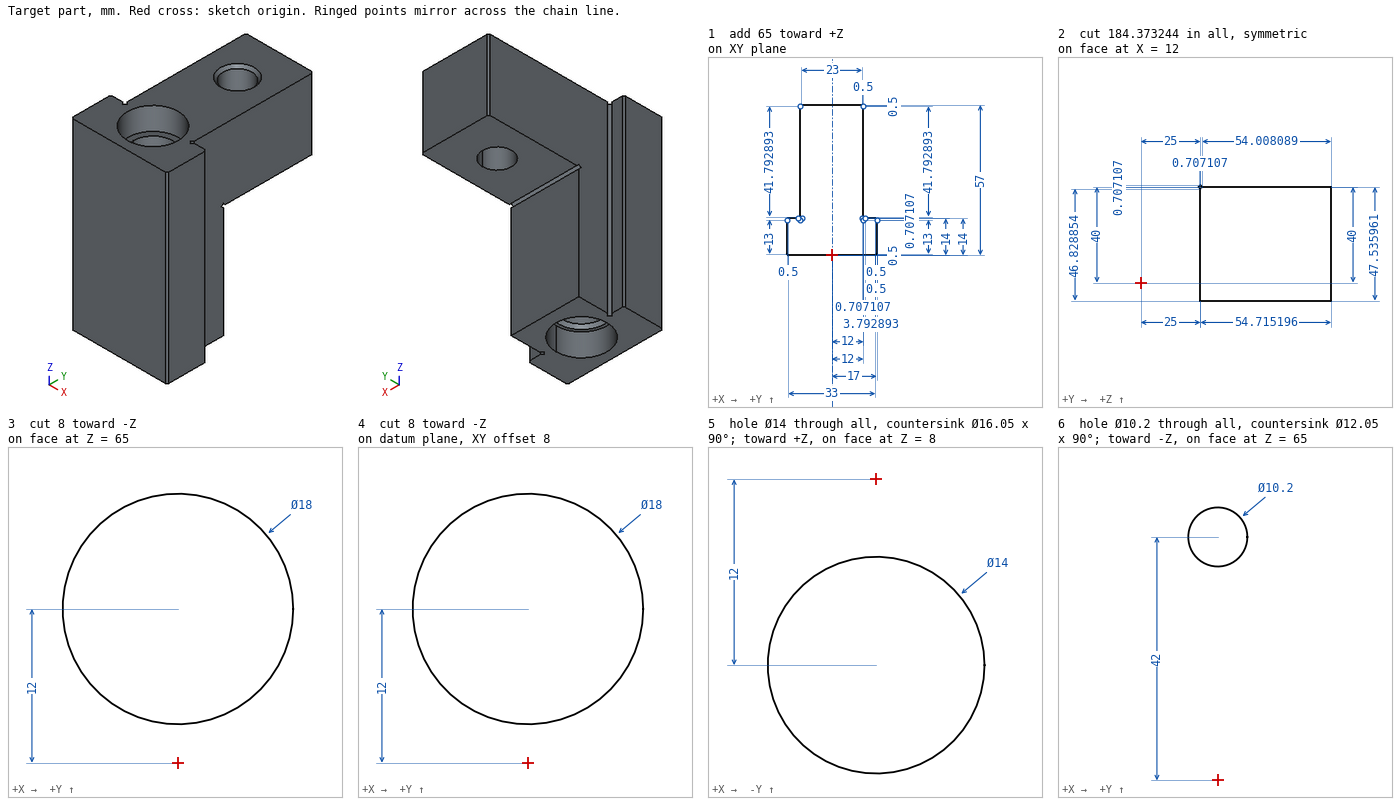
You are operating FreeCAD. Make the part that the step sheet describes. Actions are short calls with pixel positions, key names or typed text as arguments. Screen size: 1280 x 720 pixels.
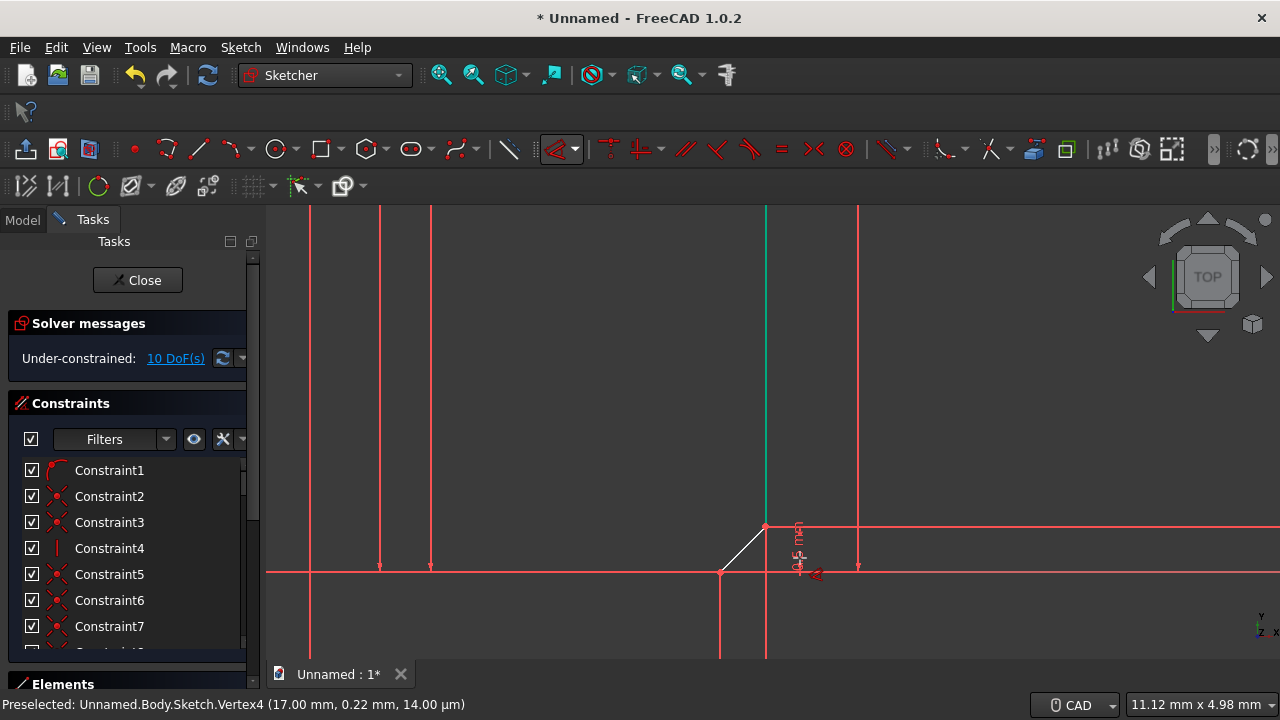
click(734, 559)
click(743, 606)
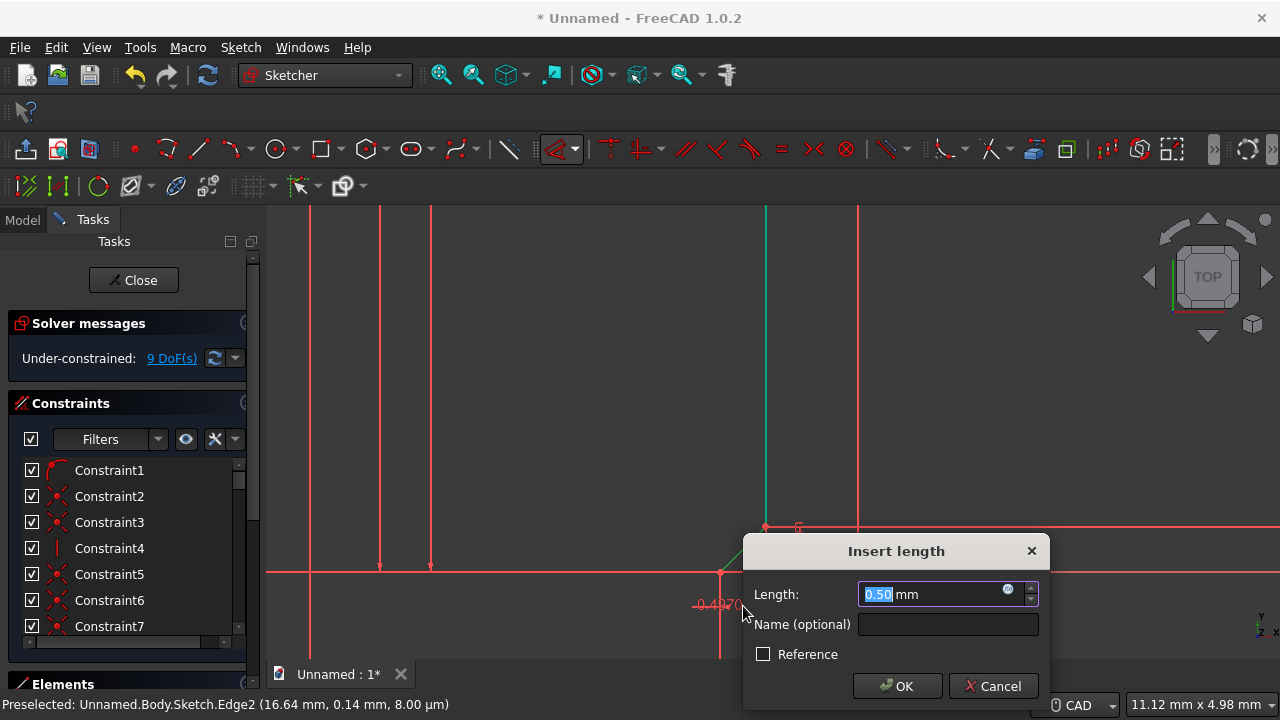
text(0.5)
key(Return)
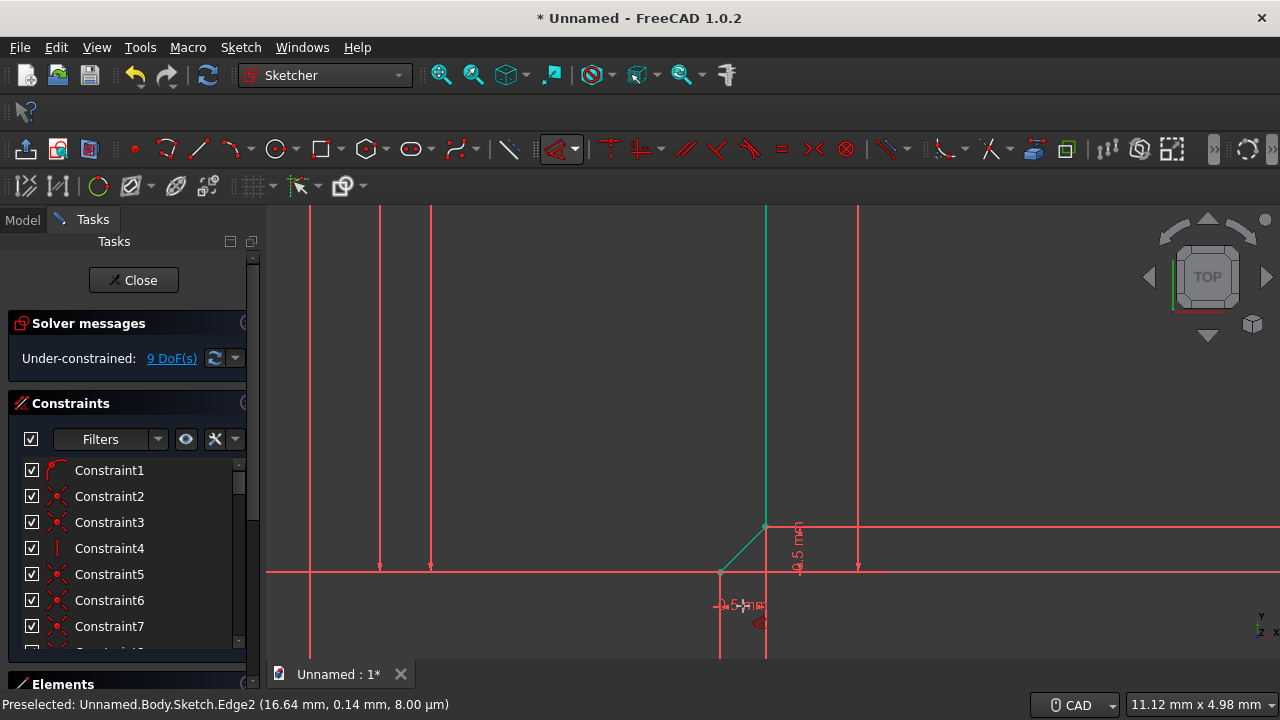
scroll(783, 561, down, 15)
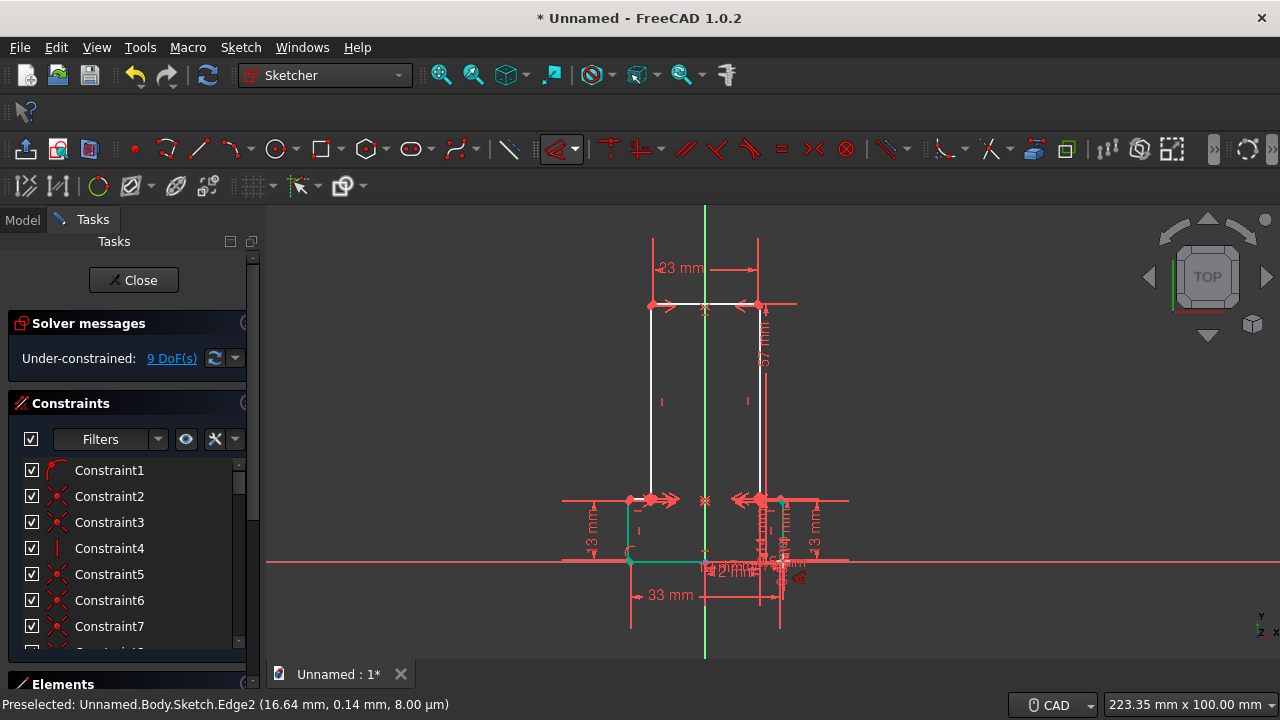
scroll(782, 500, up, 15)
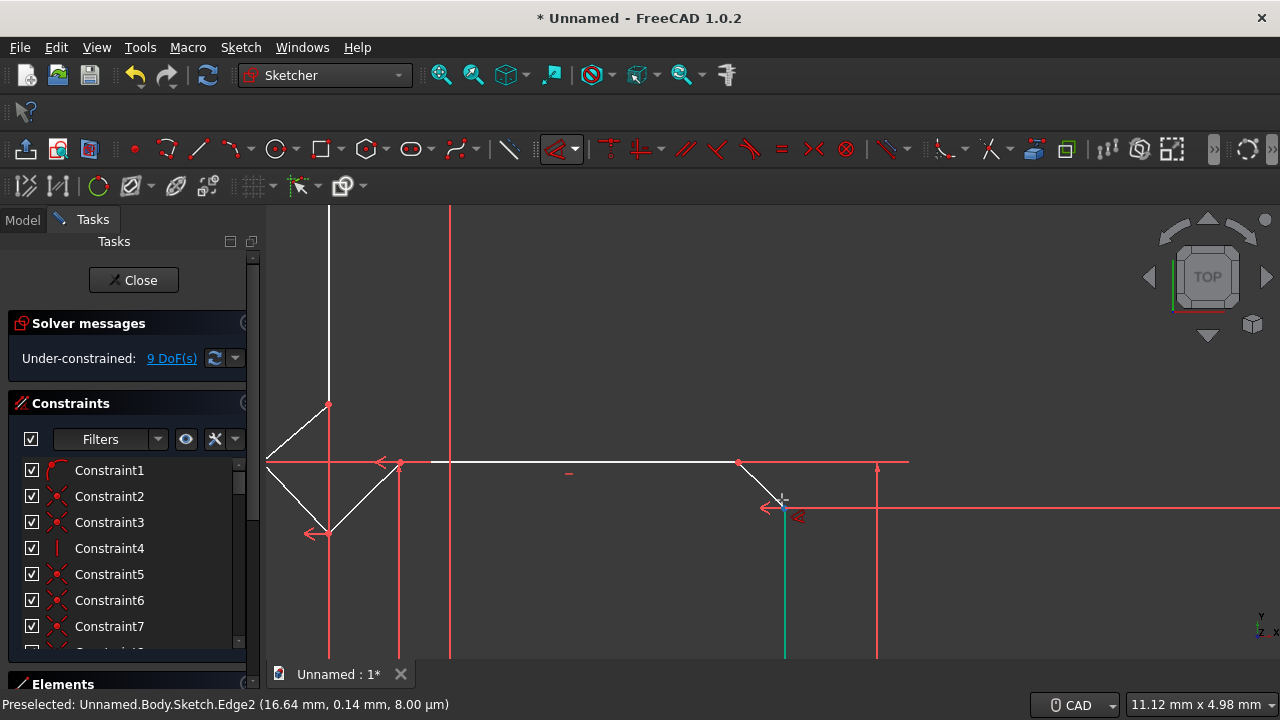
click(771, 494)
click(761, 542)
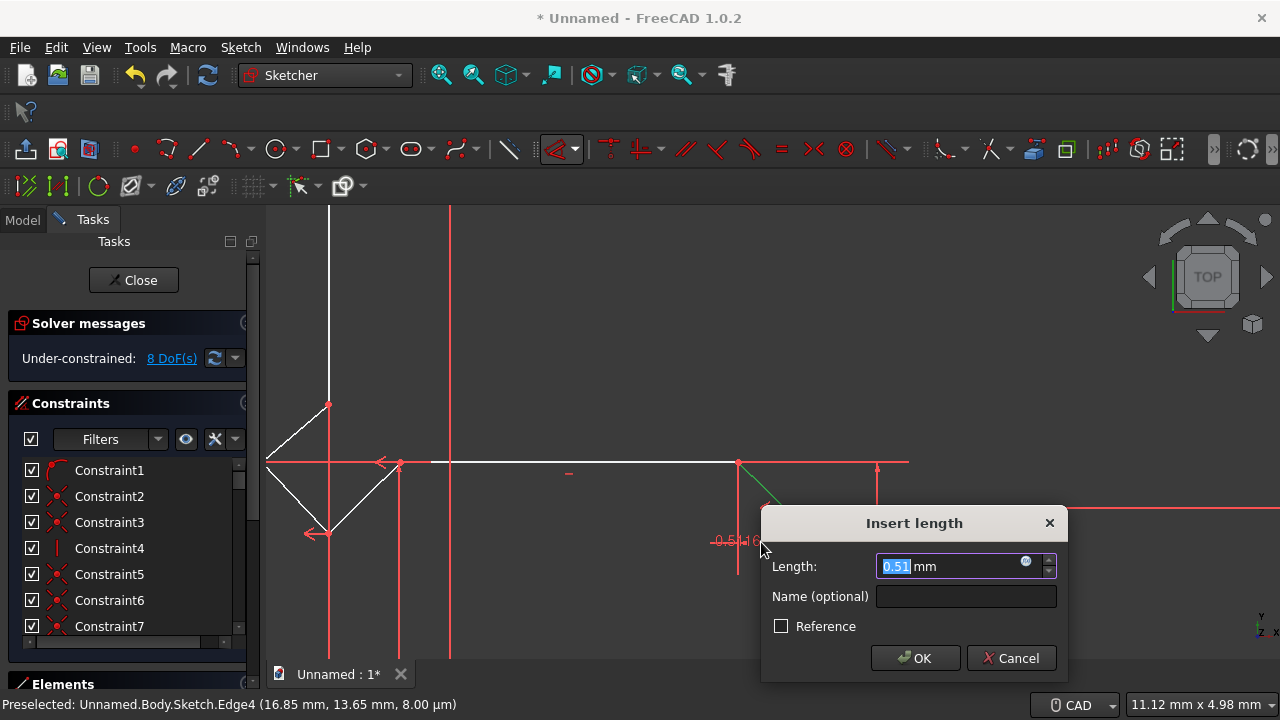
text(0.5)
key(Return)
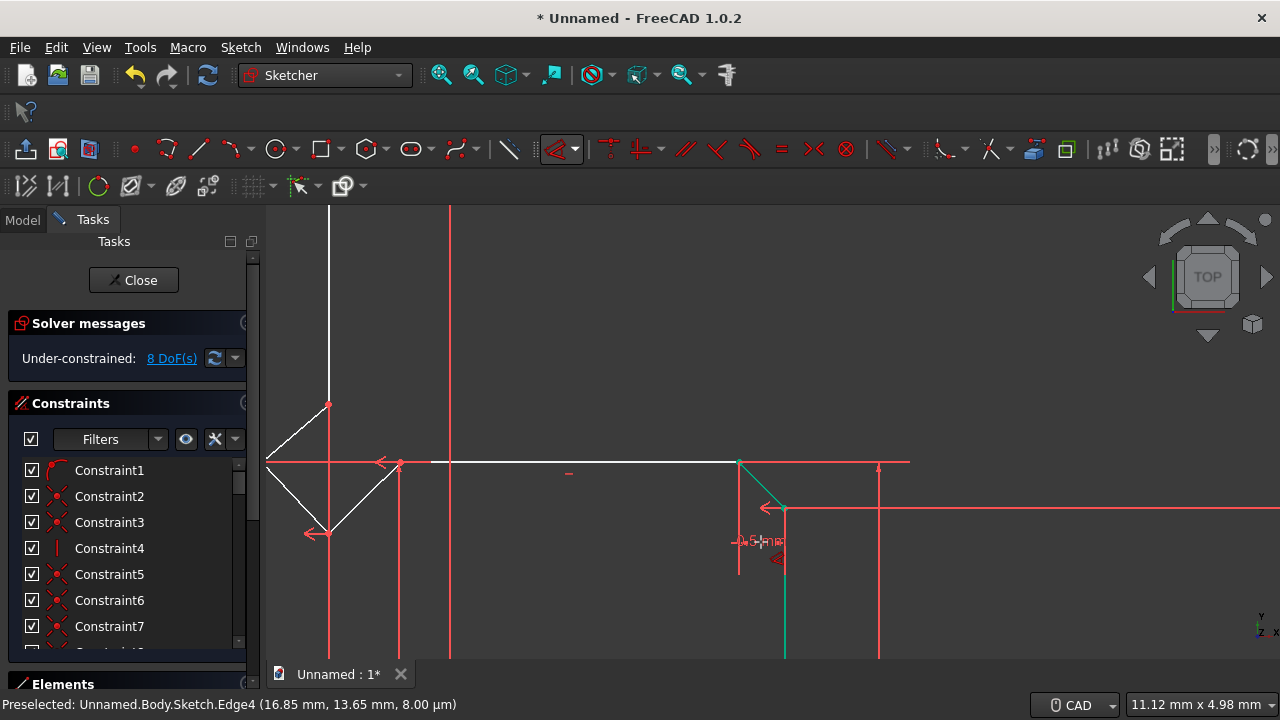
scroll(782, 500, down, 15)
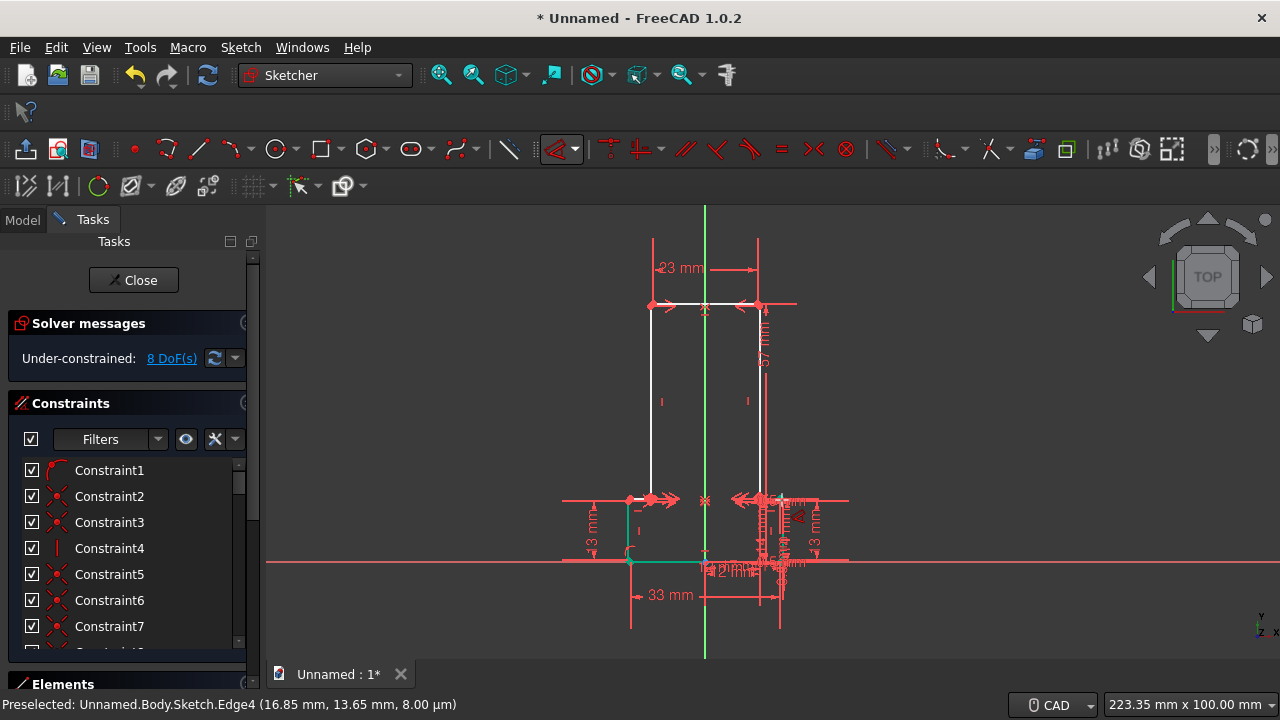
scroll(759, 305, up, 15)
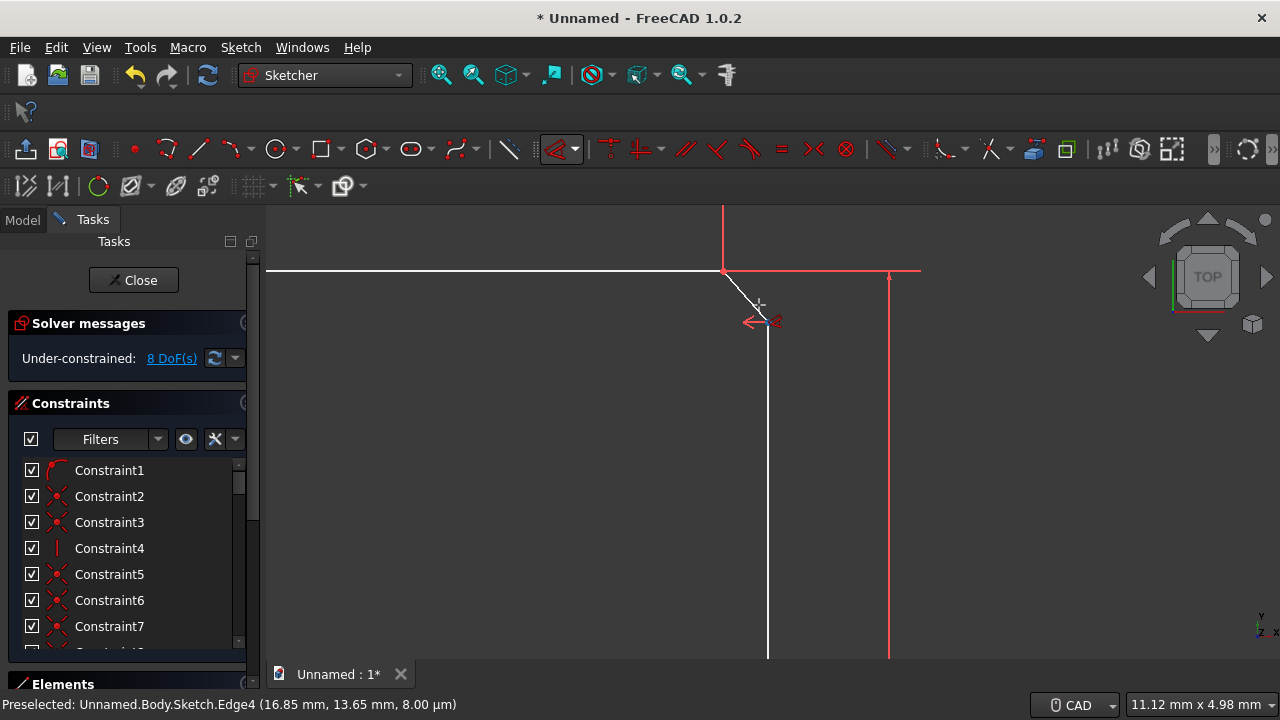
click(755, 307)
click(746, 237)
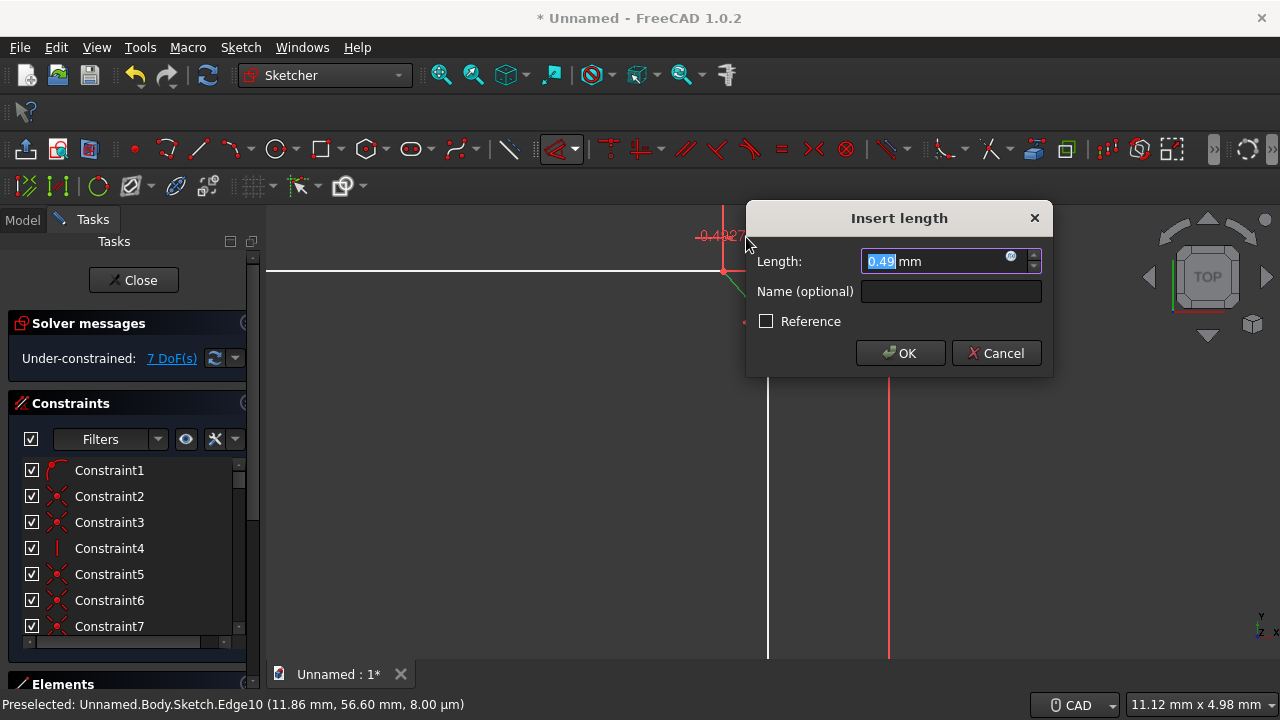
text(0.5)
key(Return)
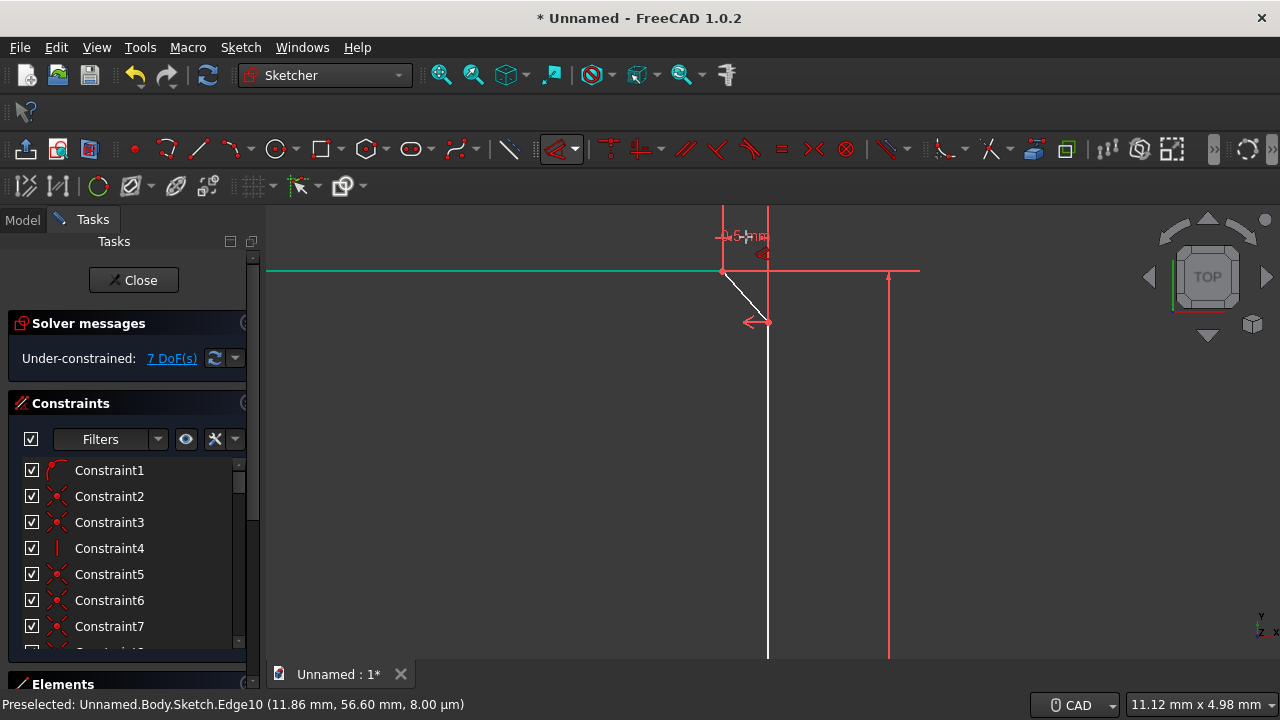
click(755, 307)
click(802, 297)